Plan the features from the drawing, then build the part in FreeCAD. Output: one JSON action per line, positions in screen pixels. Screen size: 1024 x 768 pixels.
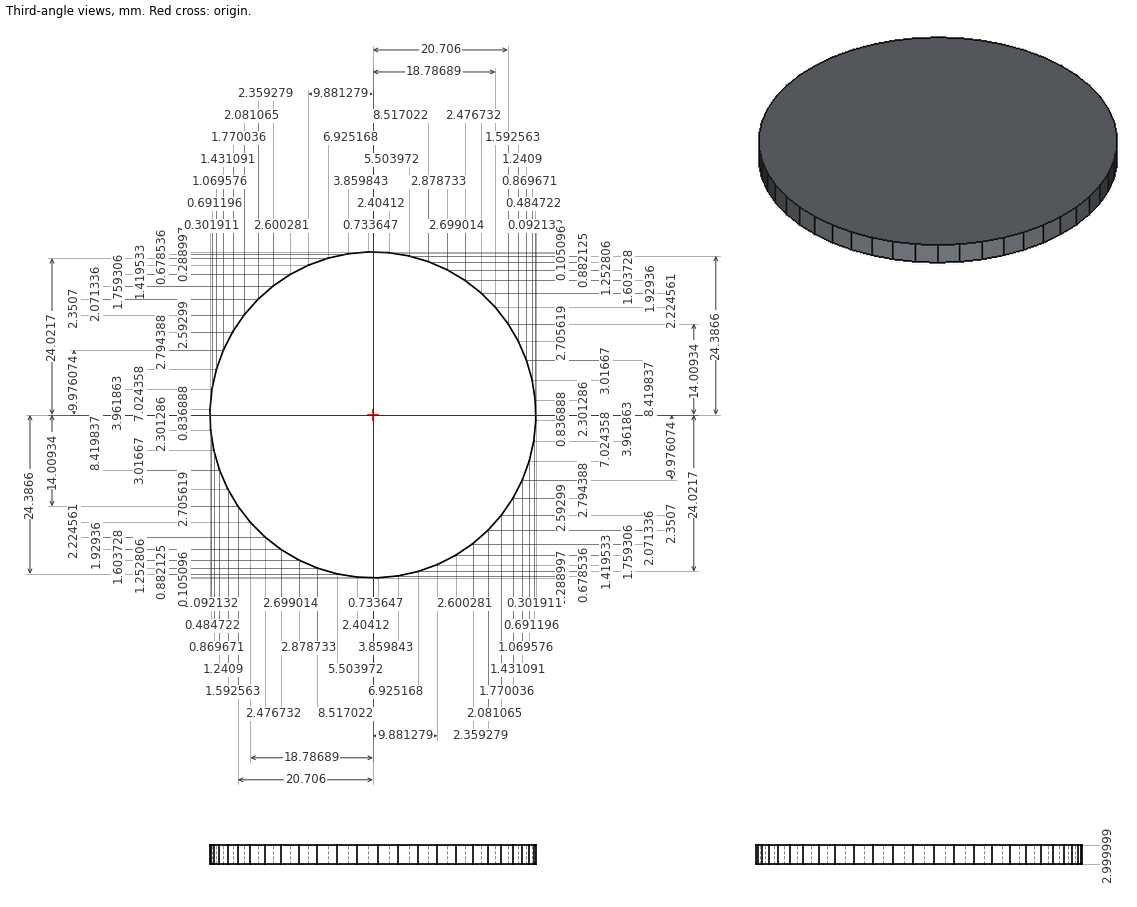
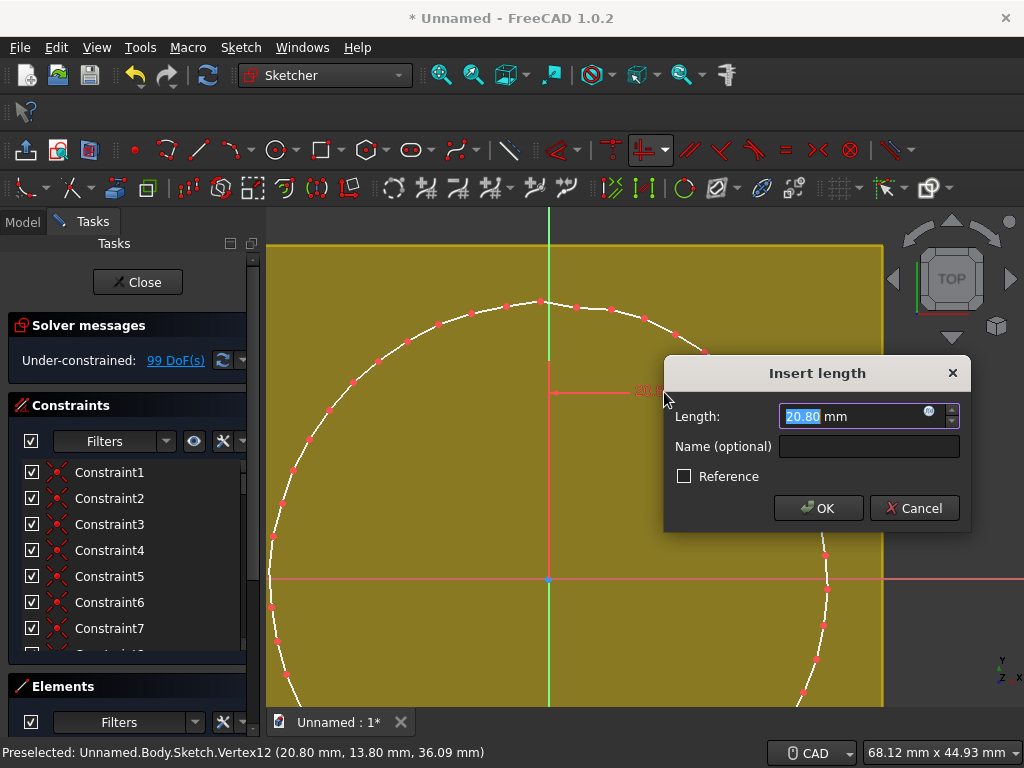
{"action": "type", "text": "20.706"}
{"action": "key", "text": "Return"}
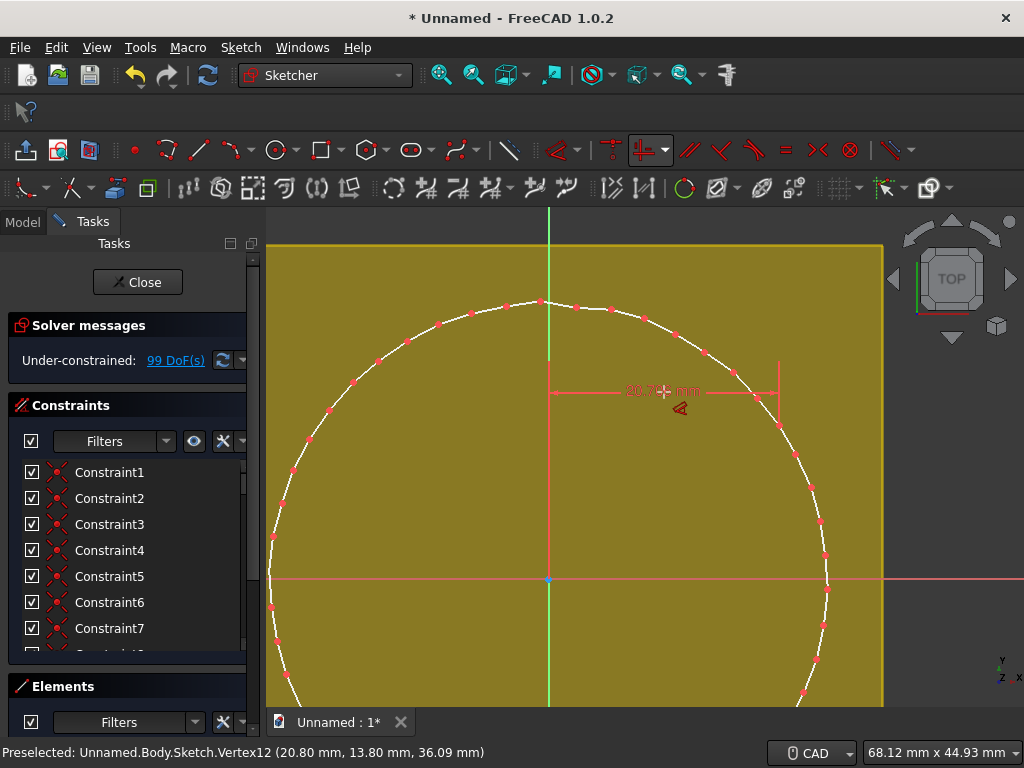
{"action": "scroll", "coordinate": [610, 309], "scroll_direction": "down", "scroll_amount": 3}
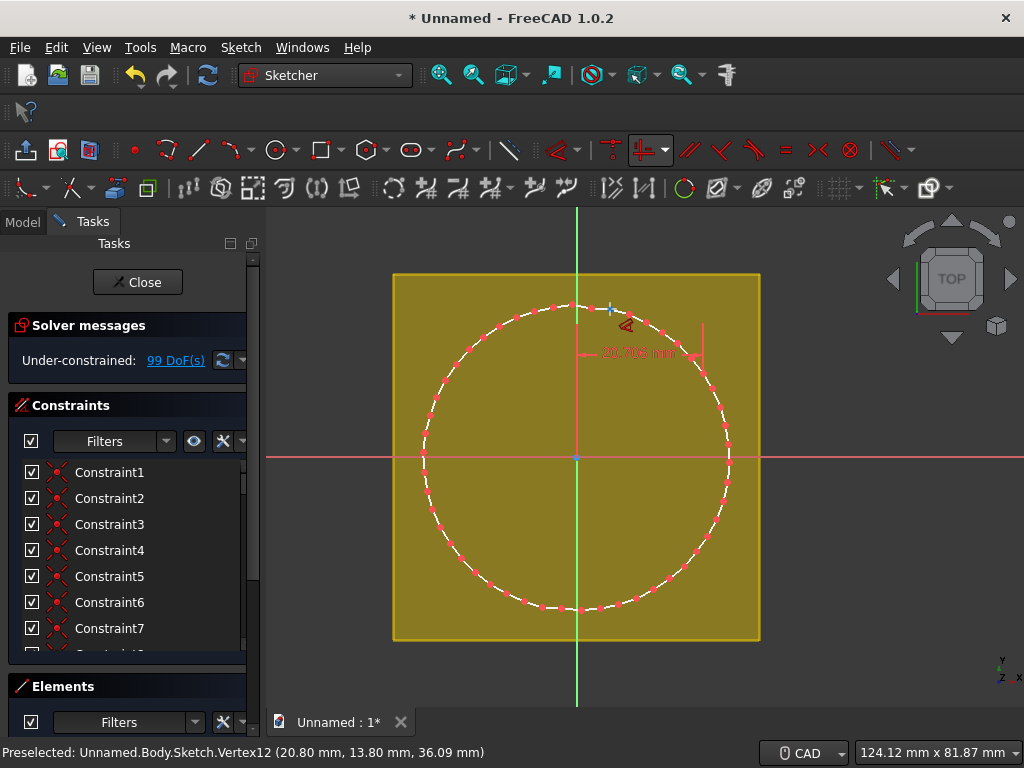
{"action": "left_click", "coordinate": [451, 544]}
{"action": "left_click", "coordinate": [514, 578]}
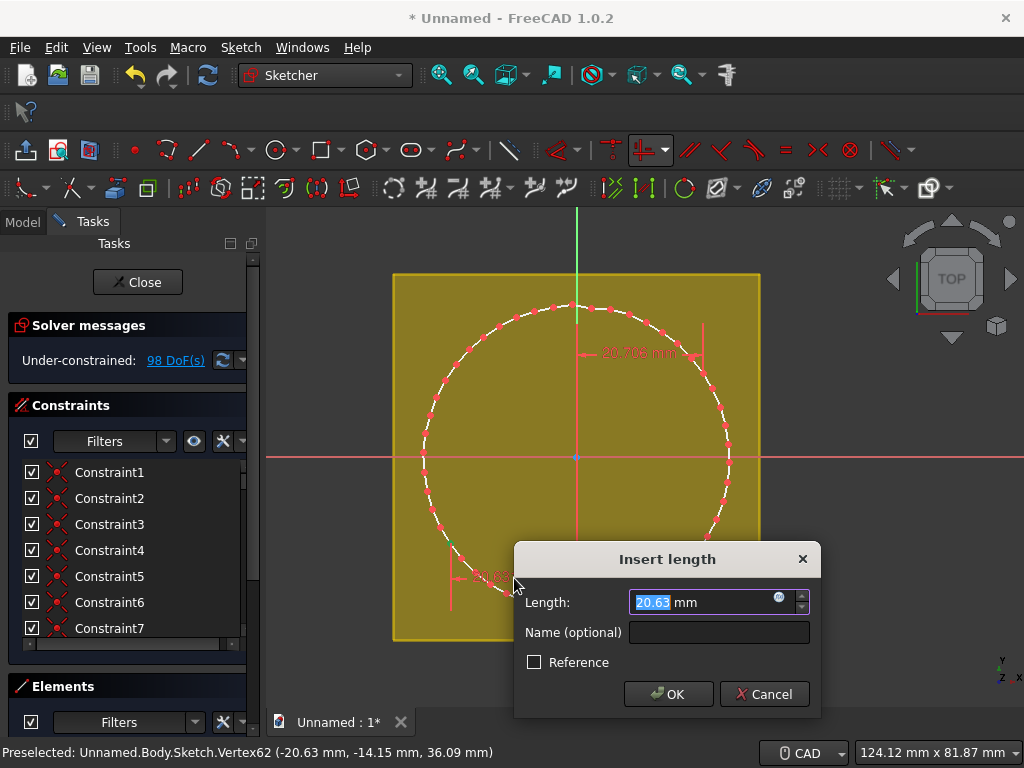
{"action": "type", "text": "20.706"}
{"action": "key", "text": "Return"}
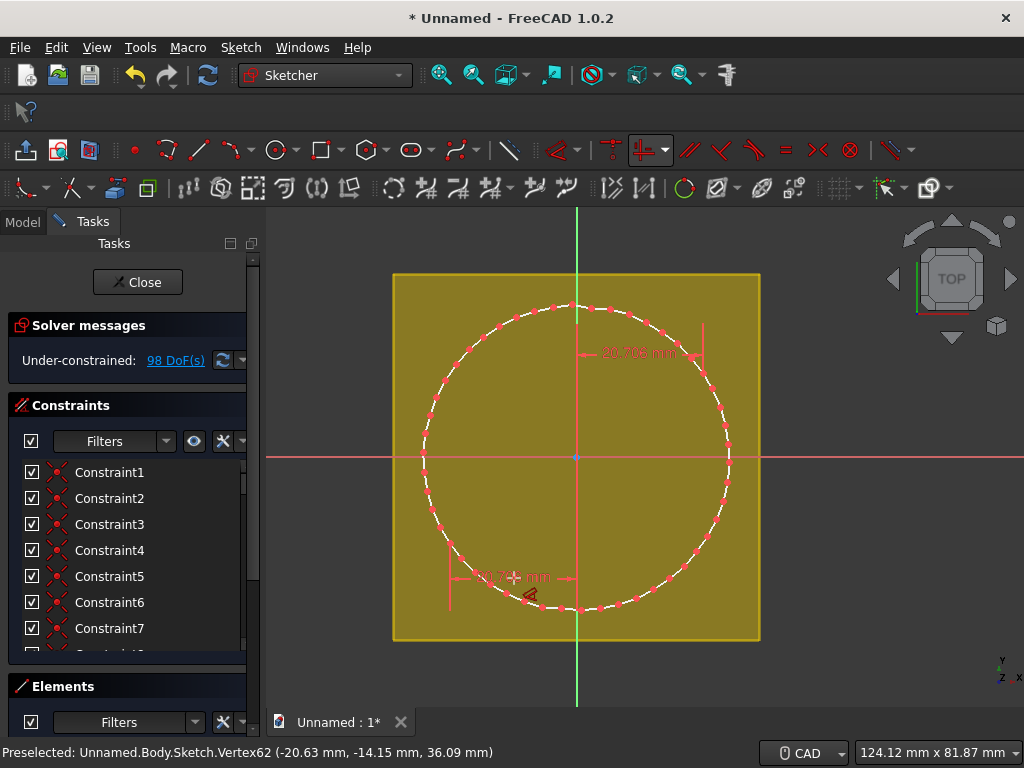
{"action": "scroll", "coordinate": [716, 398], "scroll_direction": "up", "scroll_amount": 9}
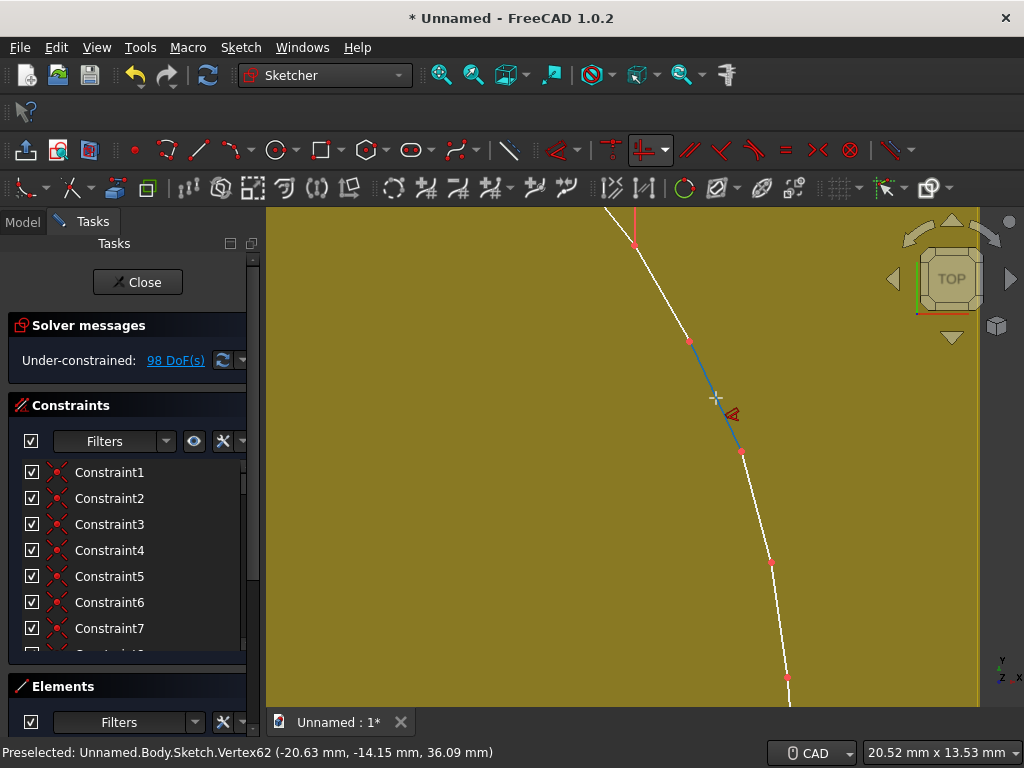
{"action": "left_click", "coordinate": [716, 396]}
{"action": "left_click", "coordinate": [716, 307]}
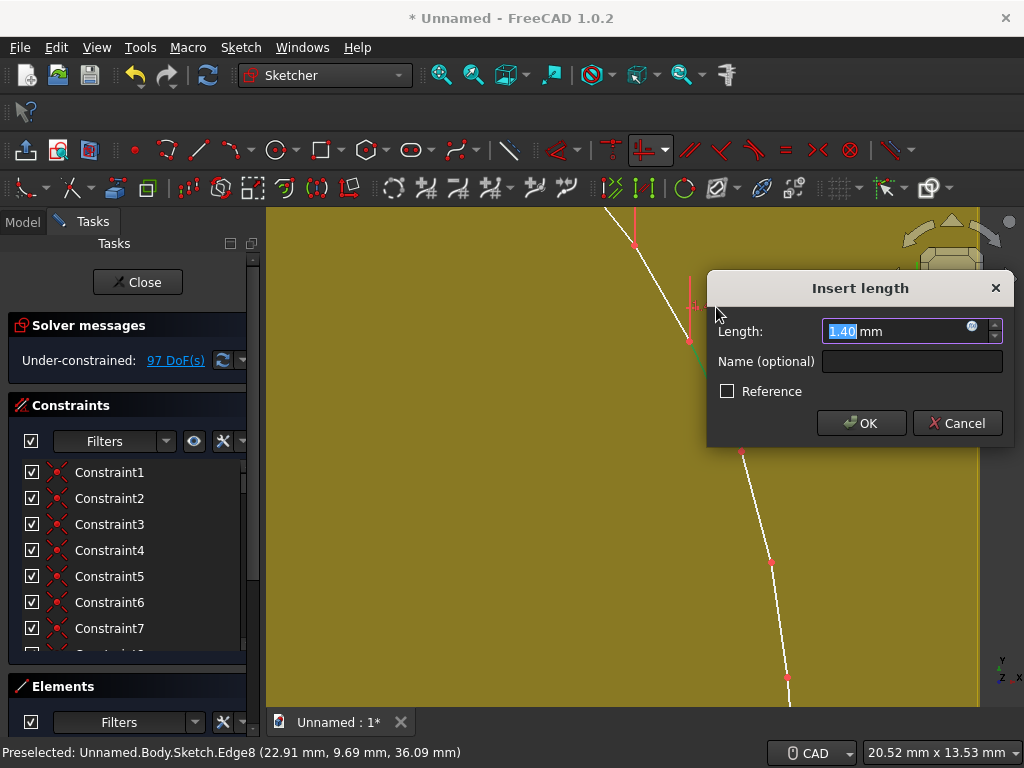
{"action": "type", "text": "1.2409"}
{"action": "key", "text": "Return"}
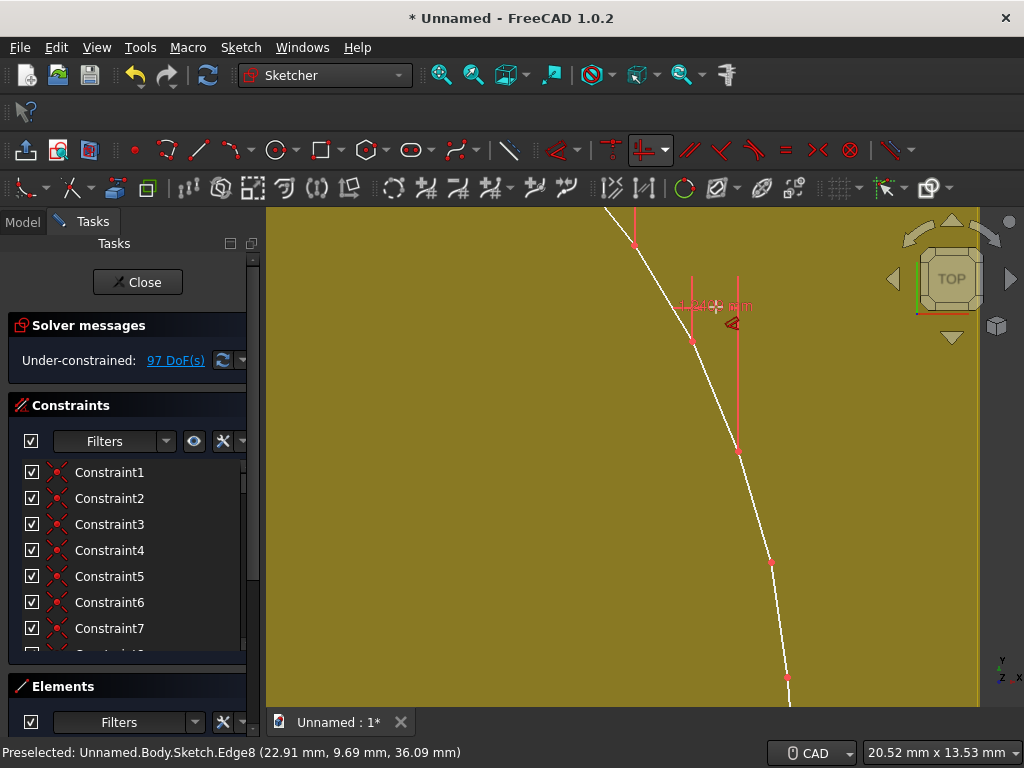
{"action": "scroll", "coordinate": [716, 398], "scroll_direction": "down", "scroll_amount": 9}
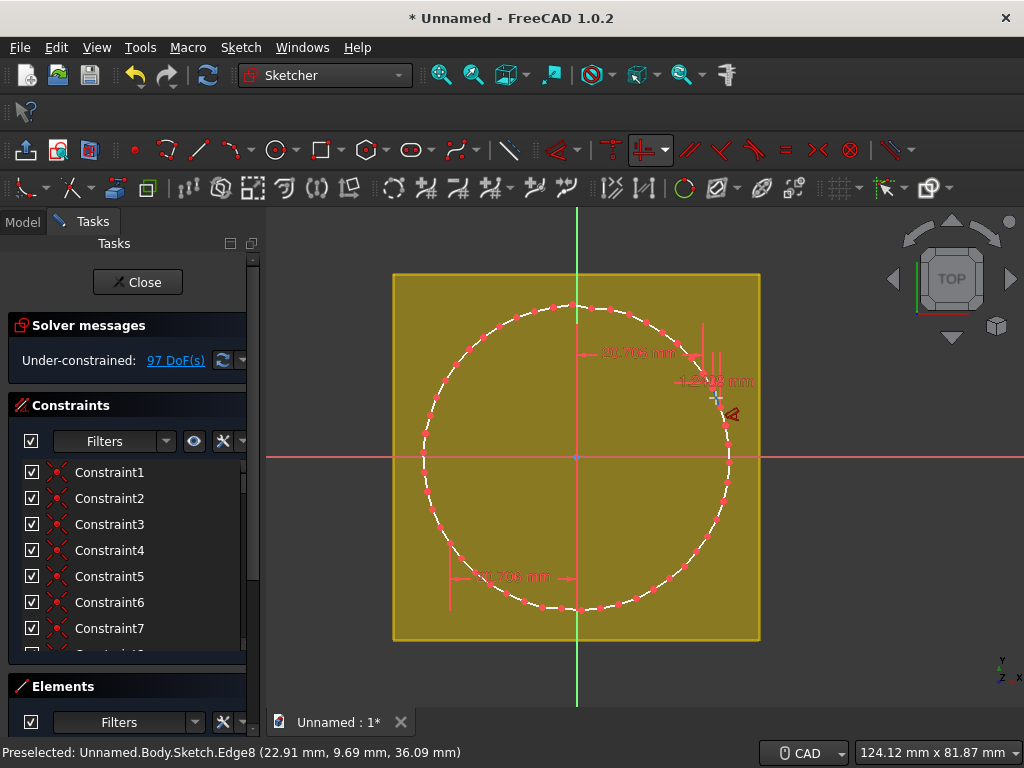
{"action": "scroll", "coordinate": [693, 556], "scroll_direction": "up", "scroll_amount": 6}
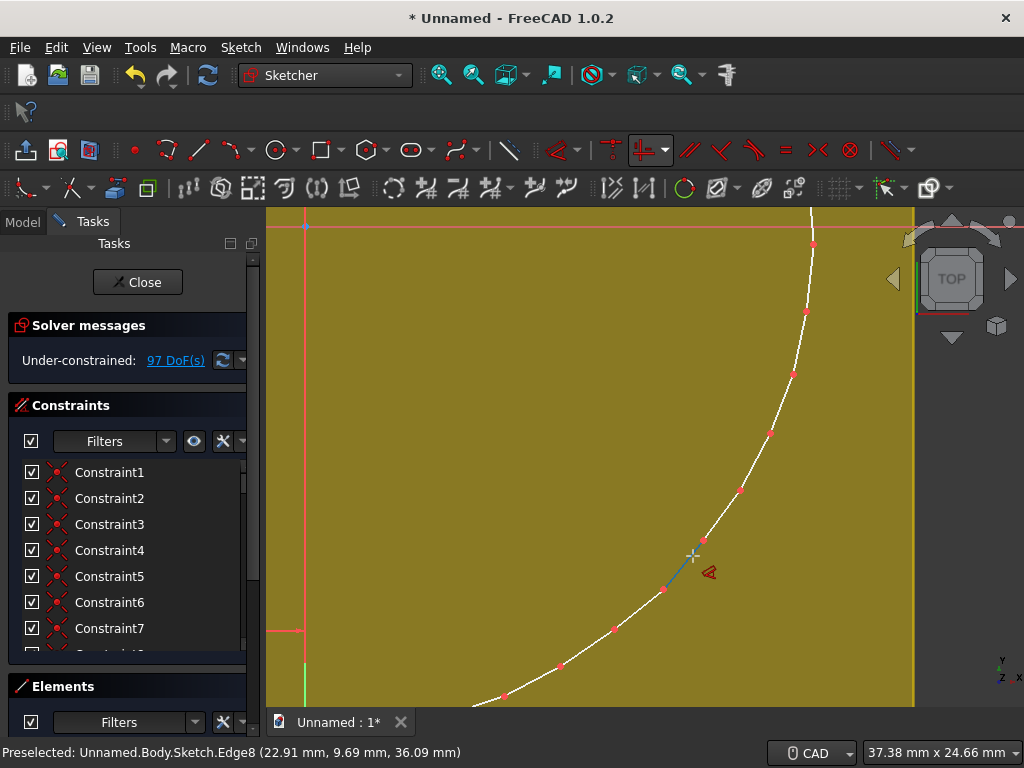
{"action": "left_click", "coordinate": [692, 555]}
{"action": "left_click", "coordinate": [738, 565]}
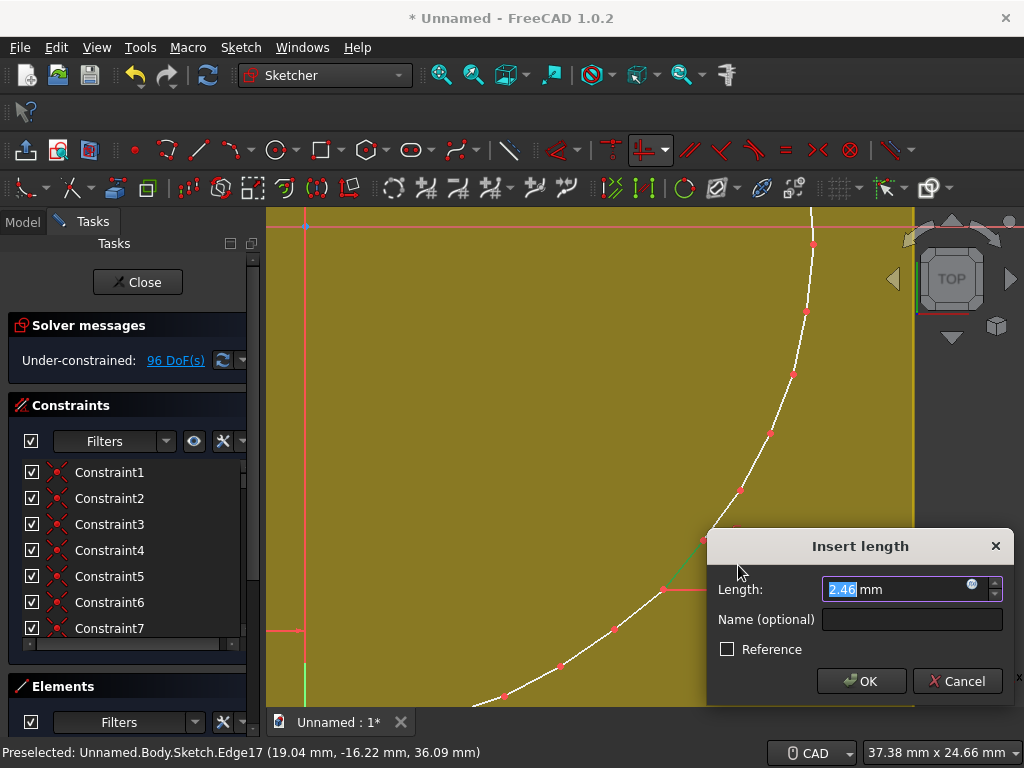
{"action": "type", "text": "2.3507"}
{"action": "key", "text": "Return"}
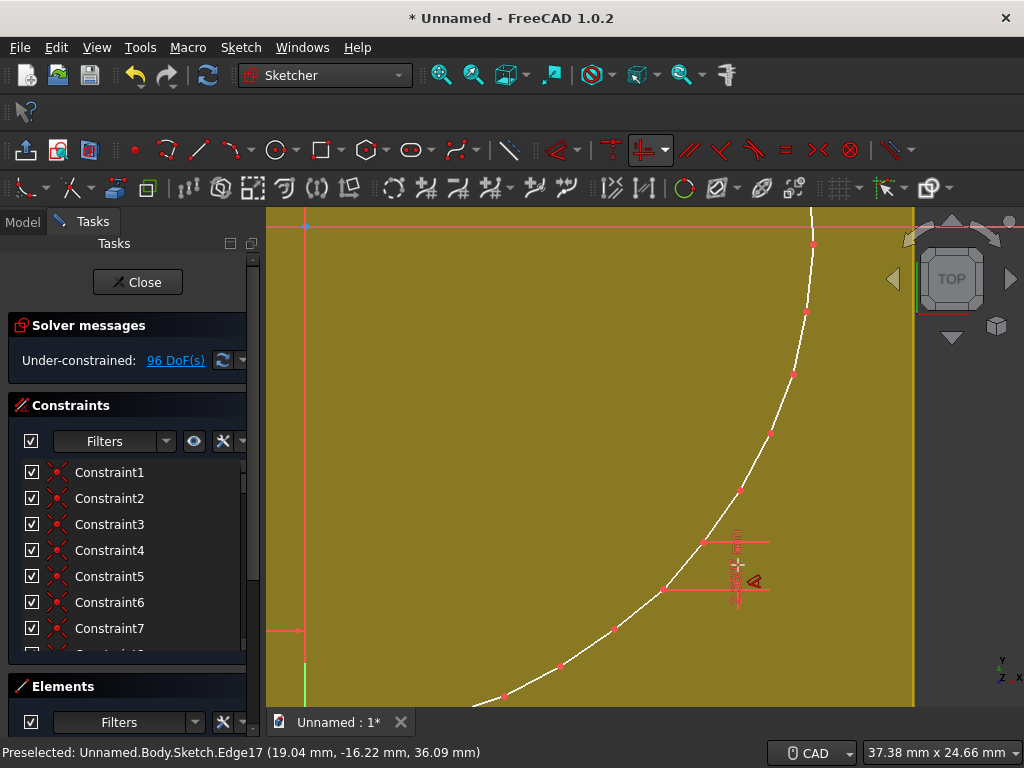
{"action": "scroll", "coordinate": [693, 556], "scroll_direction": "down", "scroll_amount": 6}